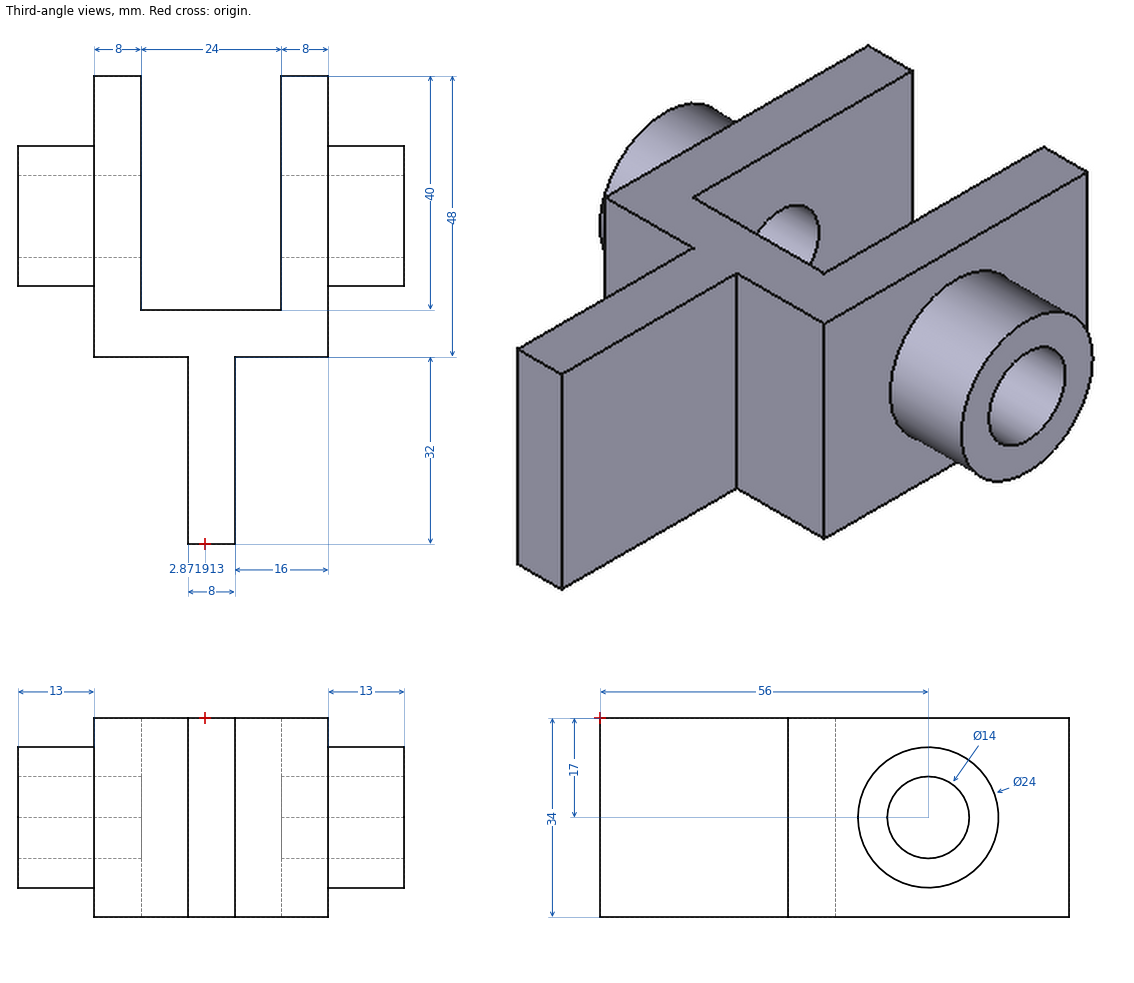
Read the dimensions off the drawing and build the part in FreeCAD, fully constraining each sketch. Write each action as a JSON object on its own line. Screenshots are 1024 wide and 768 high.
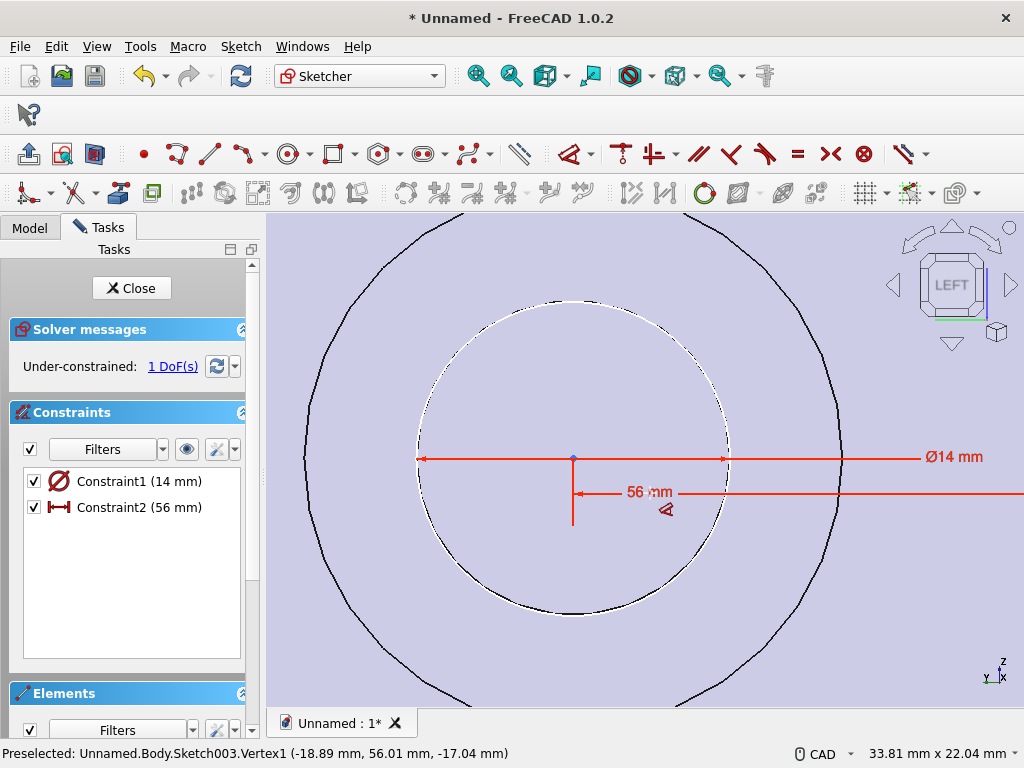
{"action": "left_click", "coordinate": [573, 459]}
{"action": "left_click", "coordinate": [539, 350]}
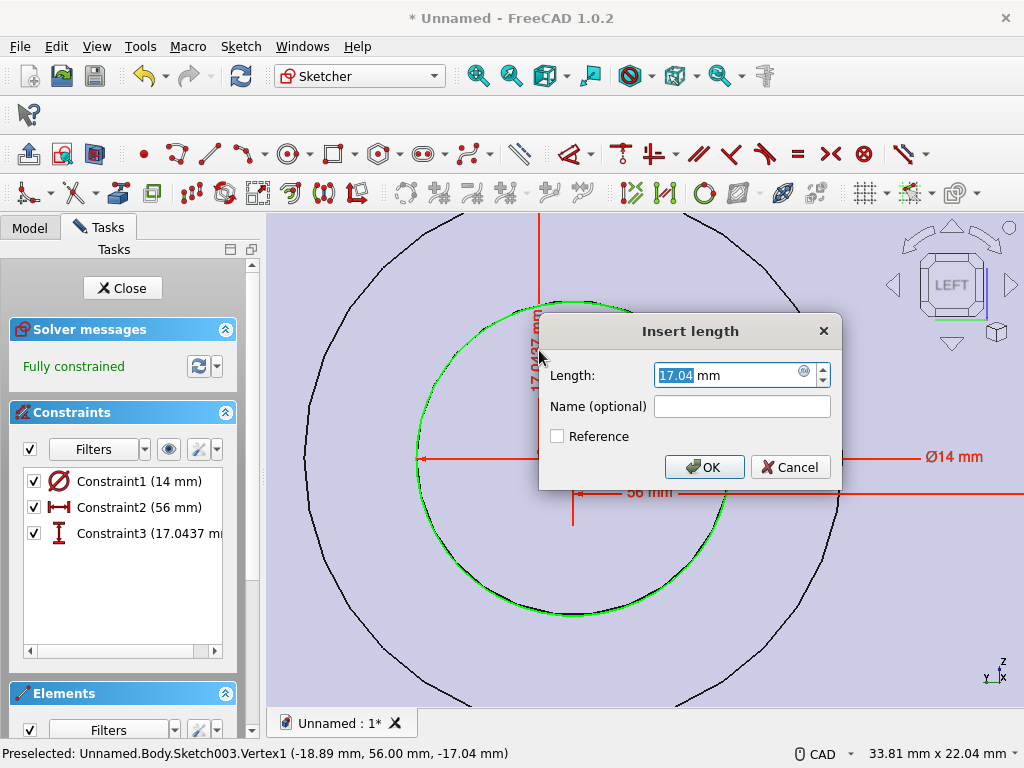
{"action": "type", "text": "17"}
{"action": "key", "text": "Return"}
{"action": "key", "text": "Escape"}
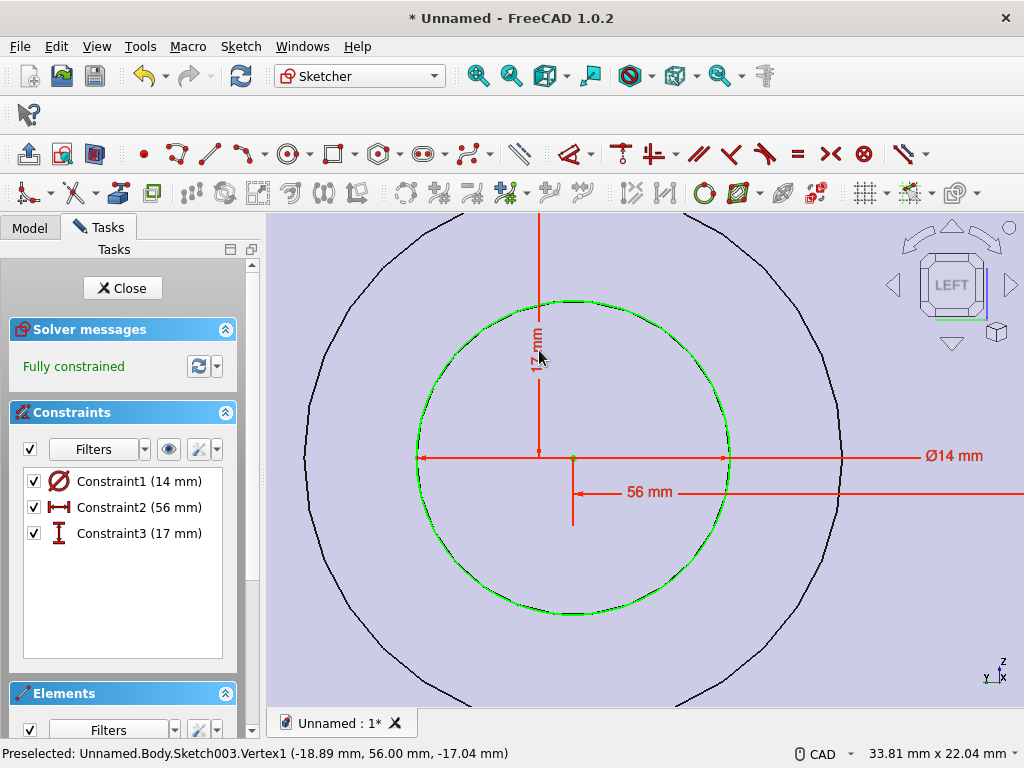
{"action": "left_click", "coordinate": [123, 288]}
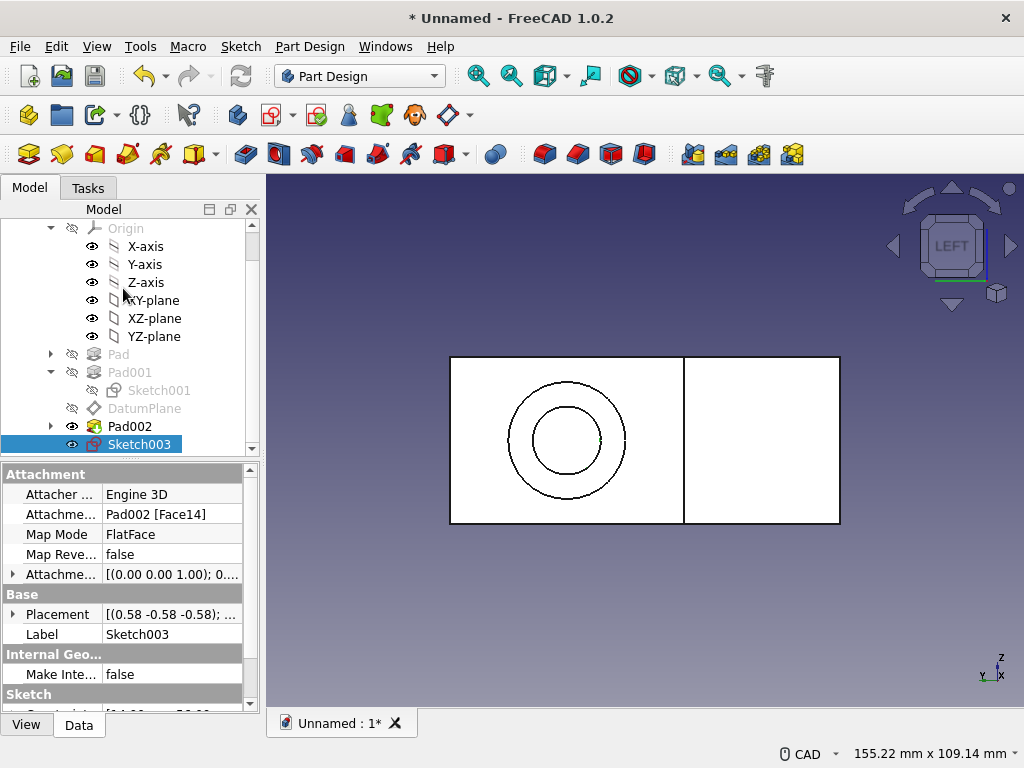
{"action": "left_click", "coordinate": [246, 154]}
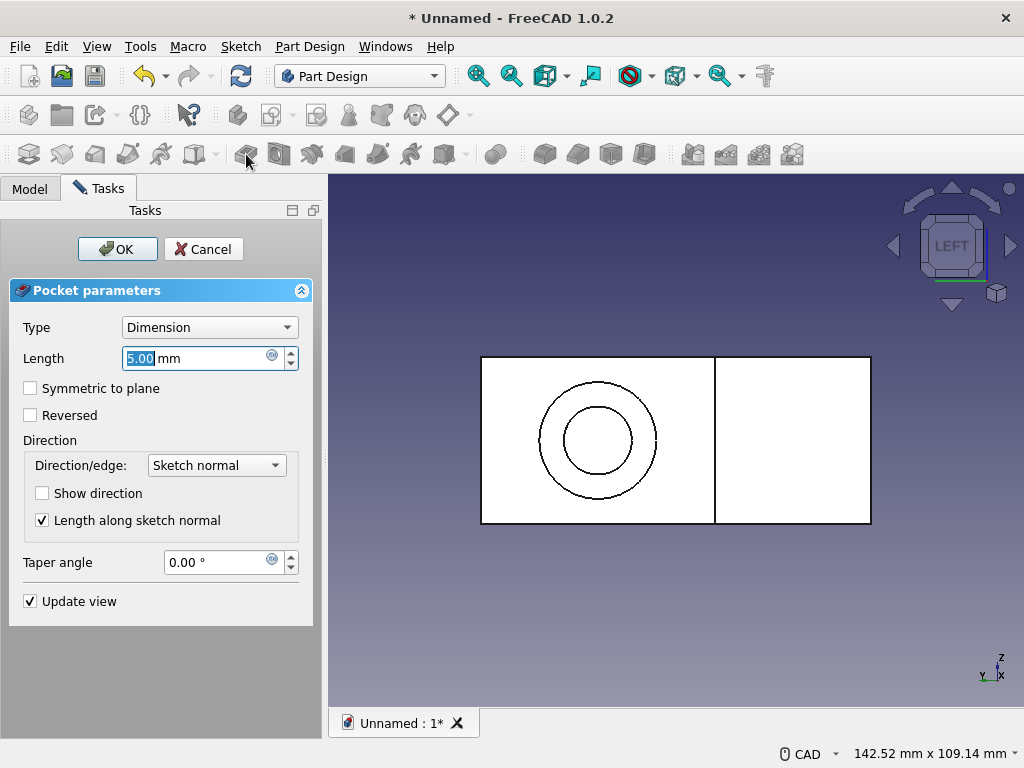
{"action": "left_click", "coordinate": [210, 328]}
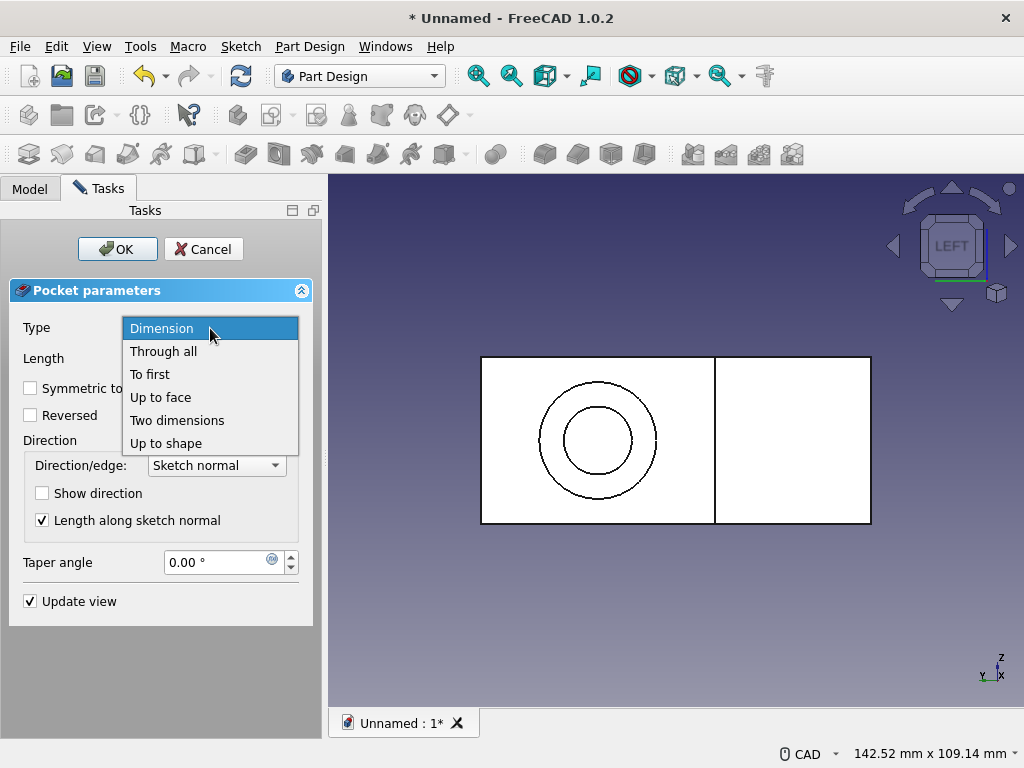
{"action": "left_click", "coordinate": [208, 352]}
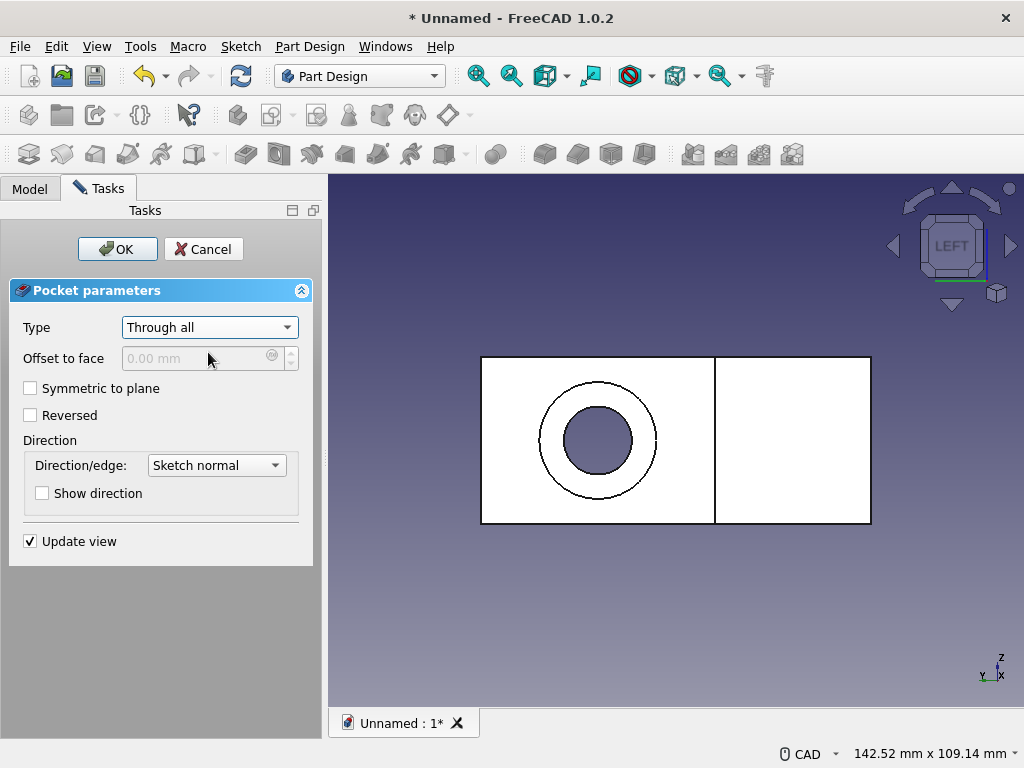
{"action": "left_click", "coordinate": [118, 249]}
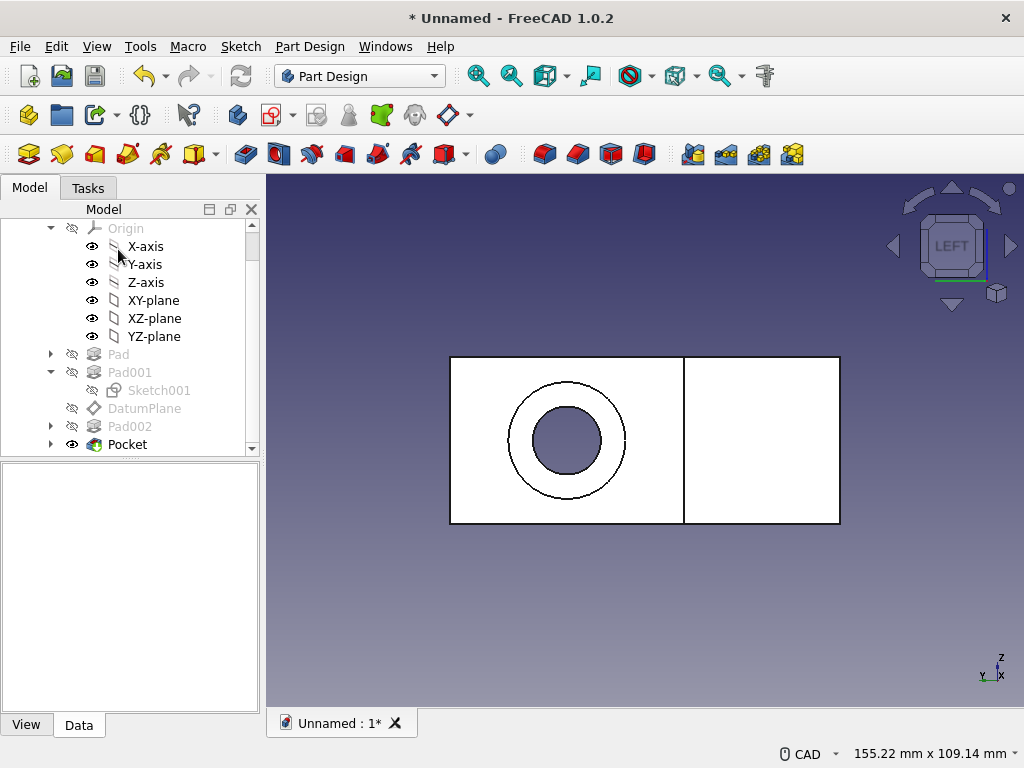
{"action": "key", "text": "0"}